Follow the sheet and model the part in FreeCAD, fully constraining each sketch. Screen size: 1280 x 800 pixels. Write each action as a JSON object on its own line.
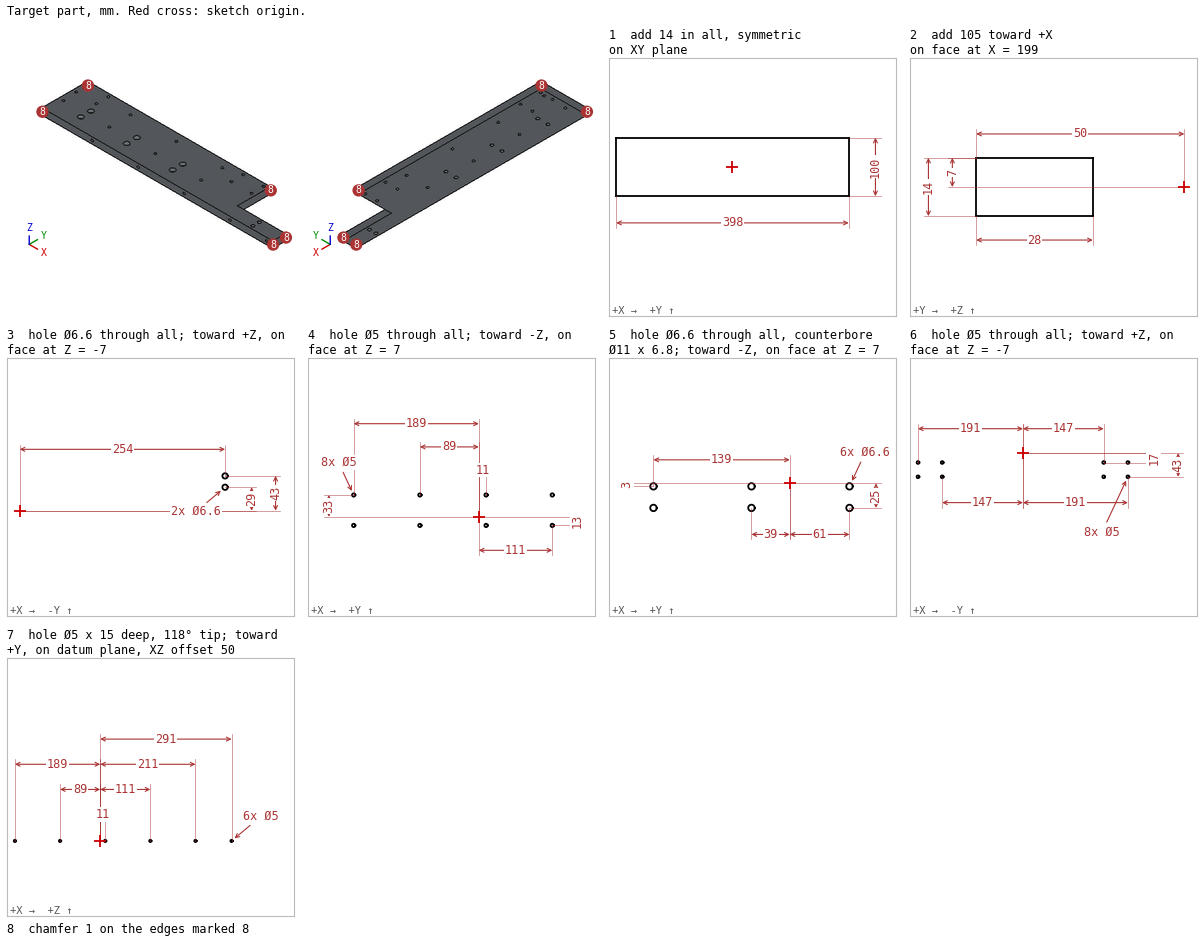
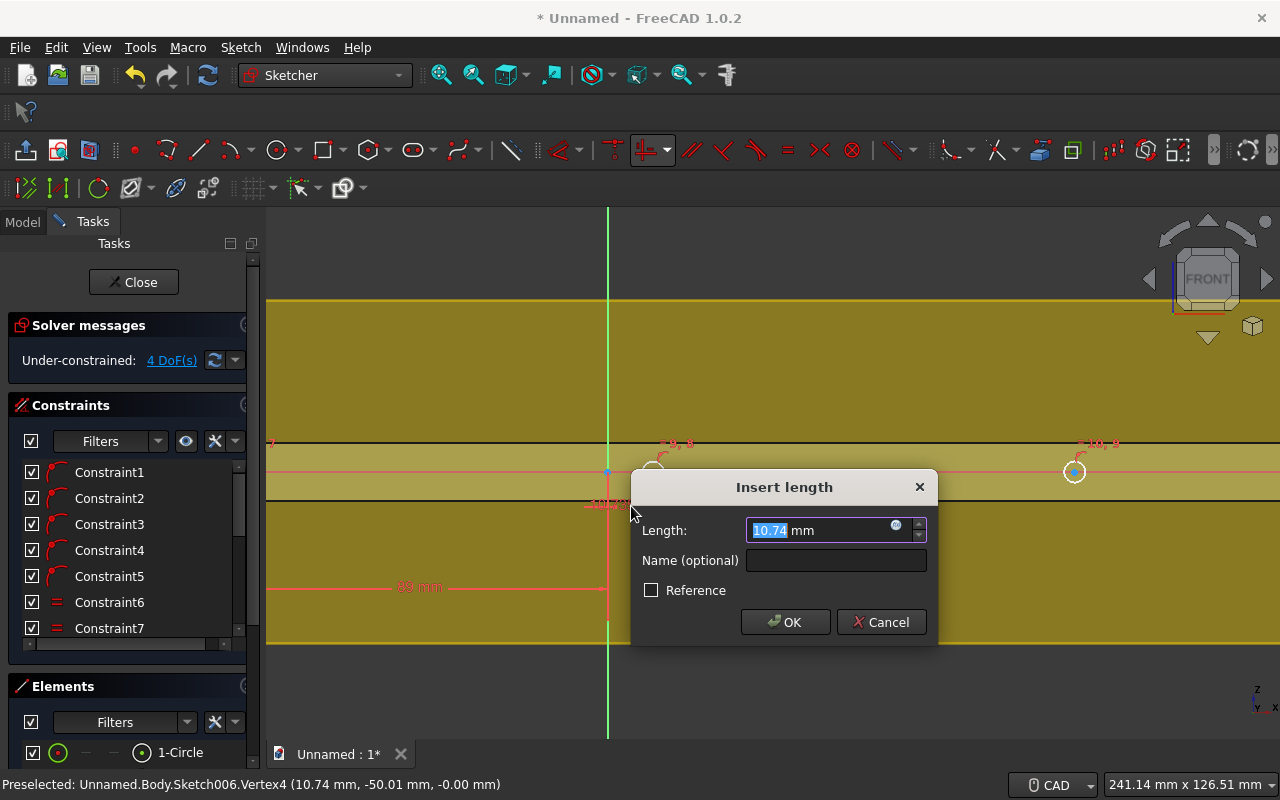
{"action": "type", "text": "11"}
{"action": "key", "text": "Return"}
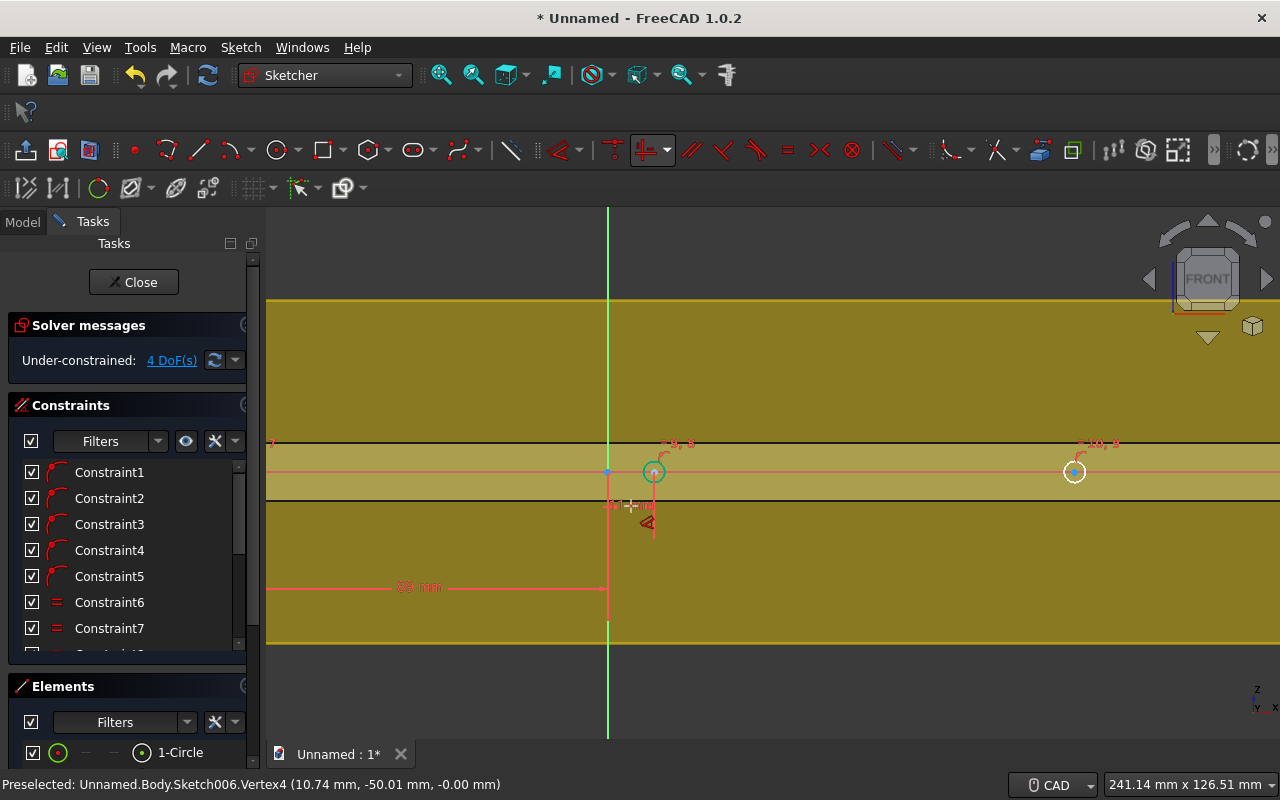
{"action": "scroll", "coordinate": [654, 473], "scroll_direction": "down", "scroll_amount": 6}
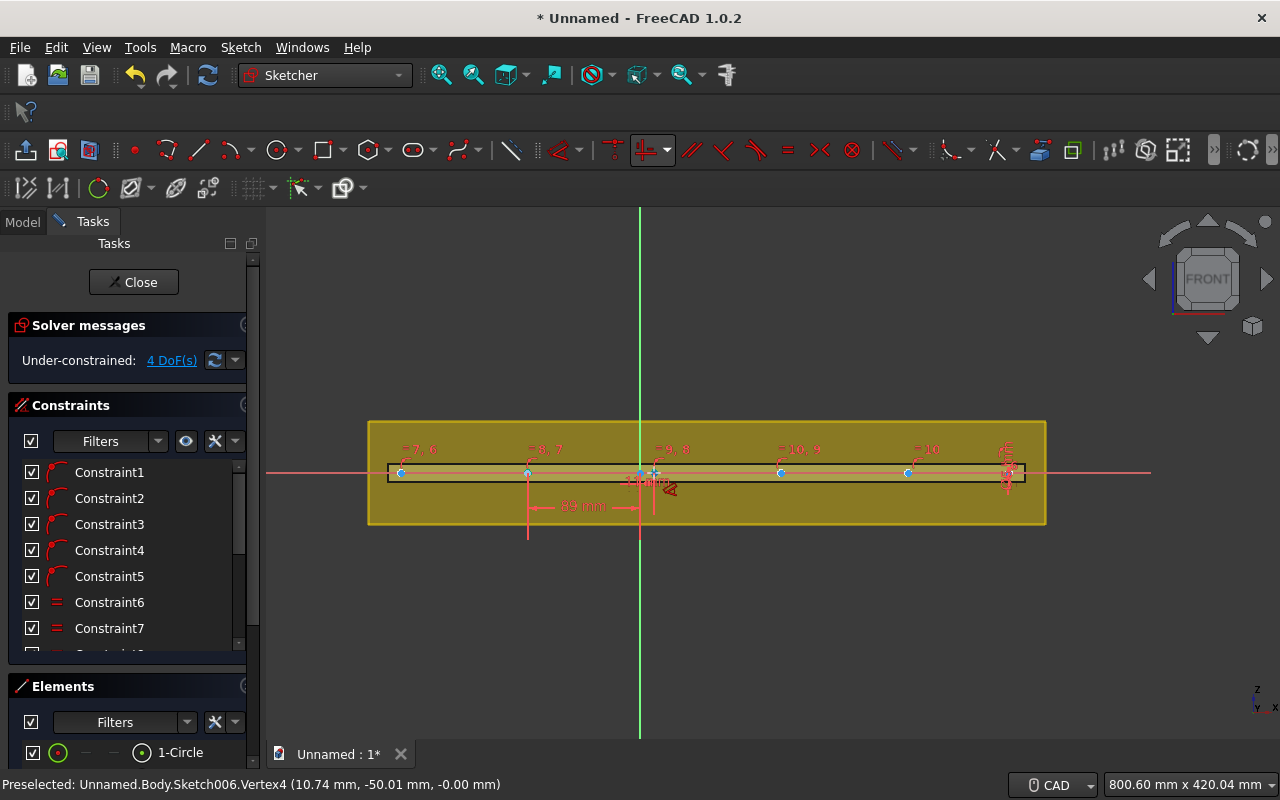
{"action": "left_click", "coordinate": [1009, 473]}
{"action": "left_click", "coordinate": [825, 507]}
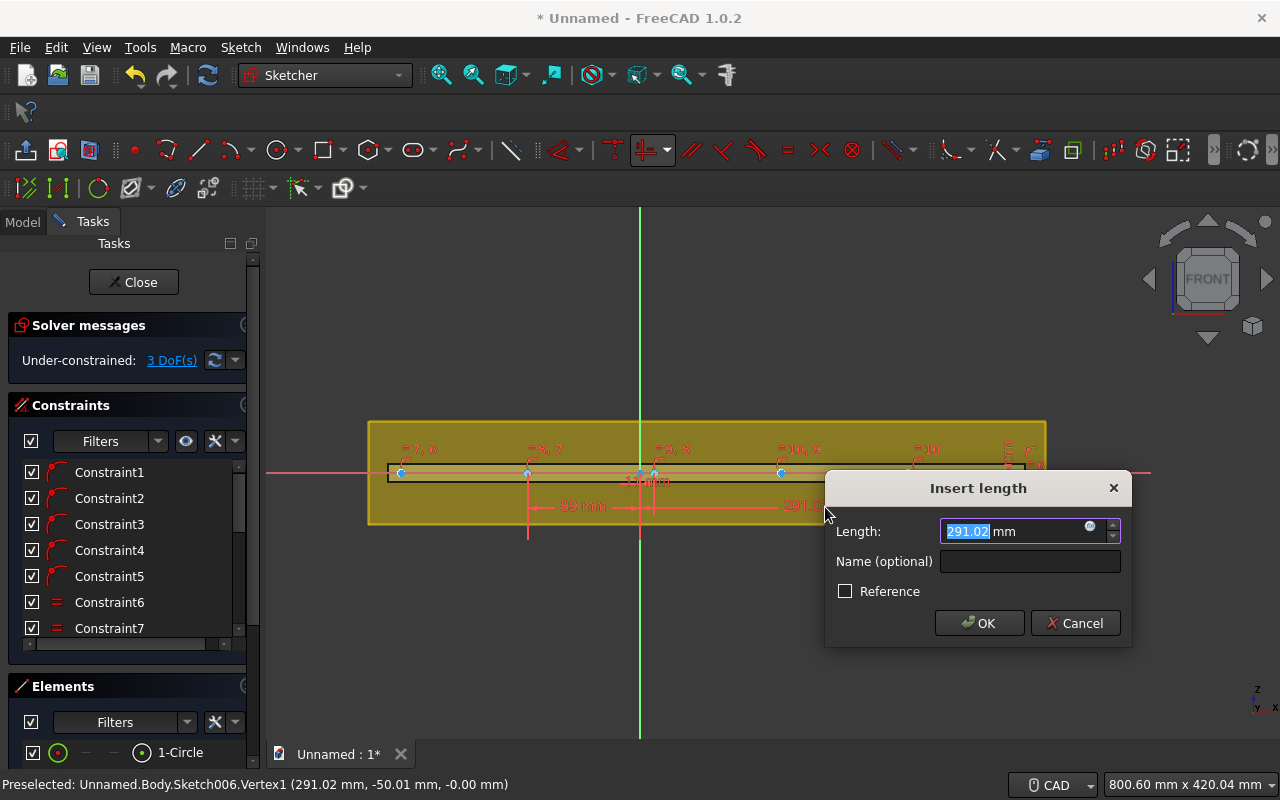
{"action": "type", "text": "291"}
{"action": "key", "text": "Return"}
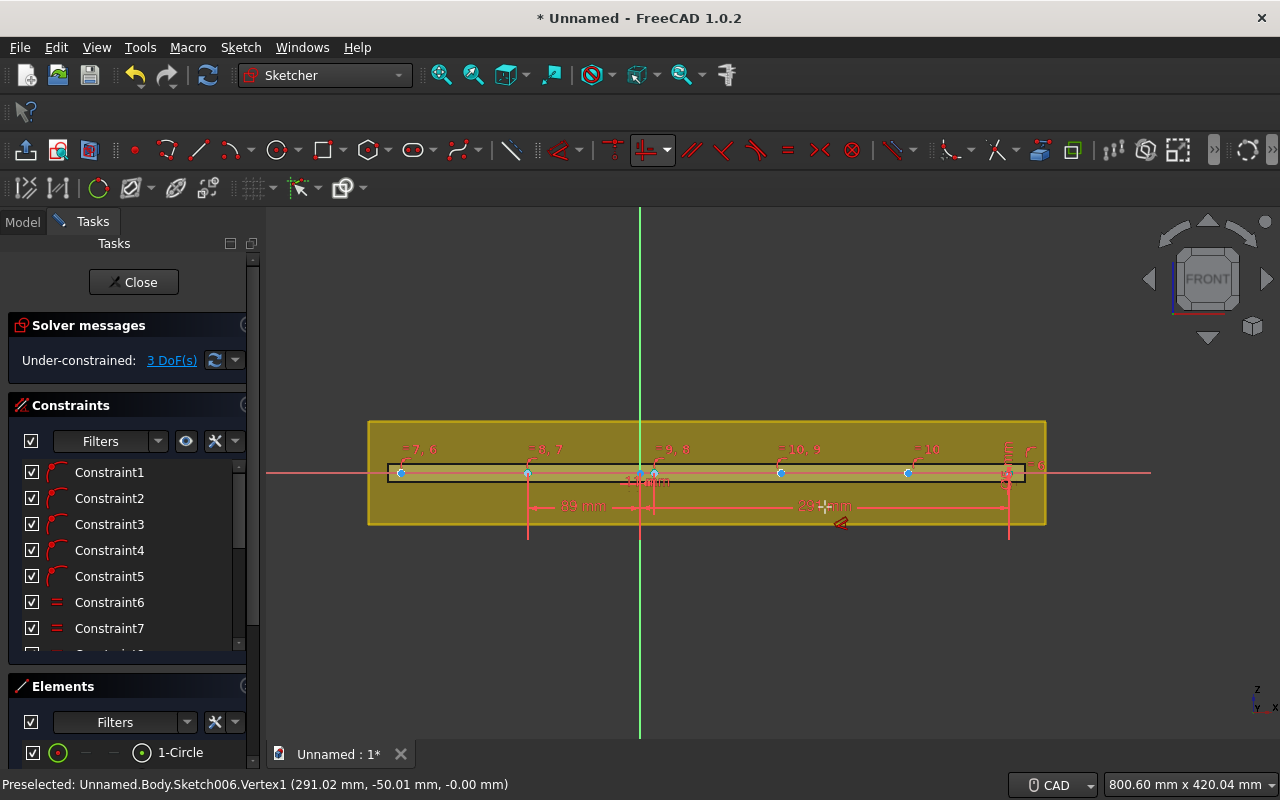
{"action": "left_click", "coordinate": [401, 473]}
{"action": "left_click", "coordinate": [466, 507]}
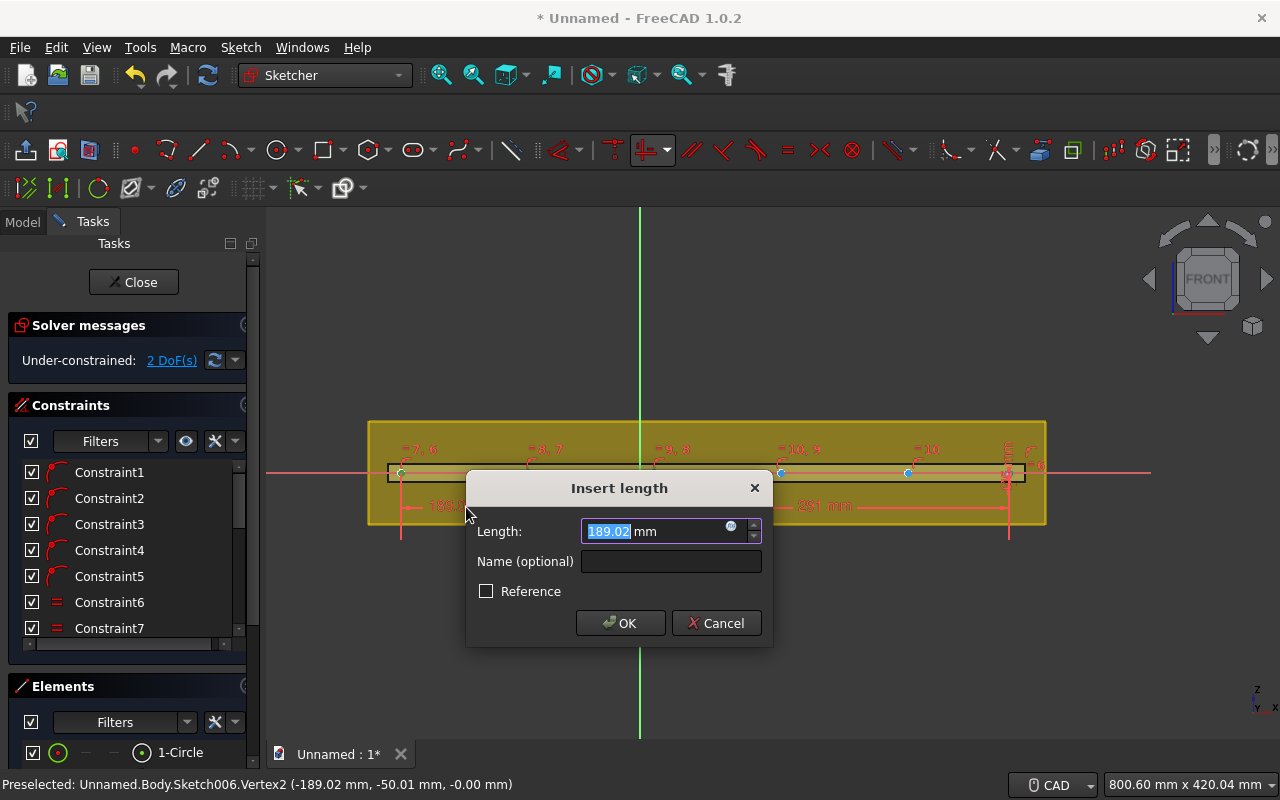
{"action": "type", "text": "189"}
{"action": "key", "text": "Return"}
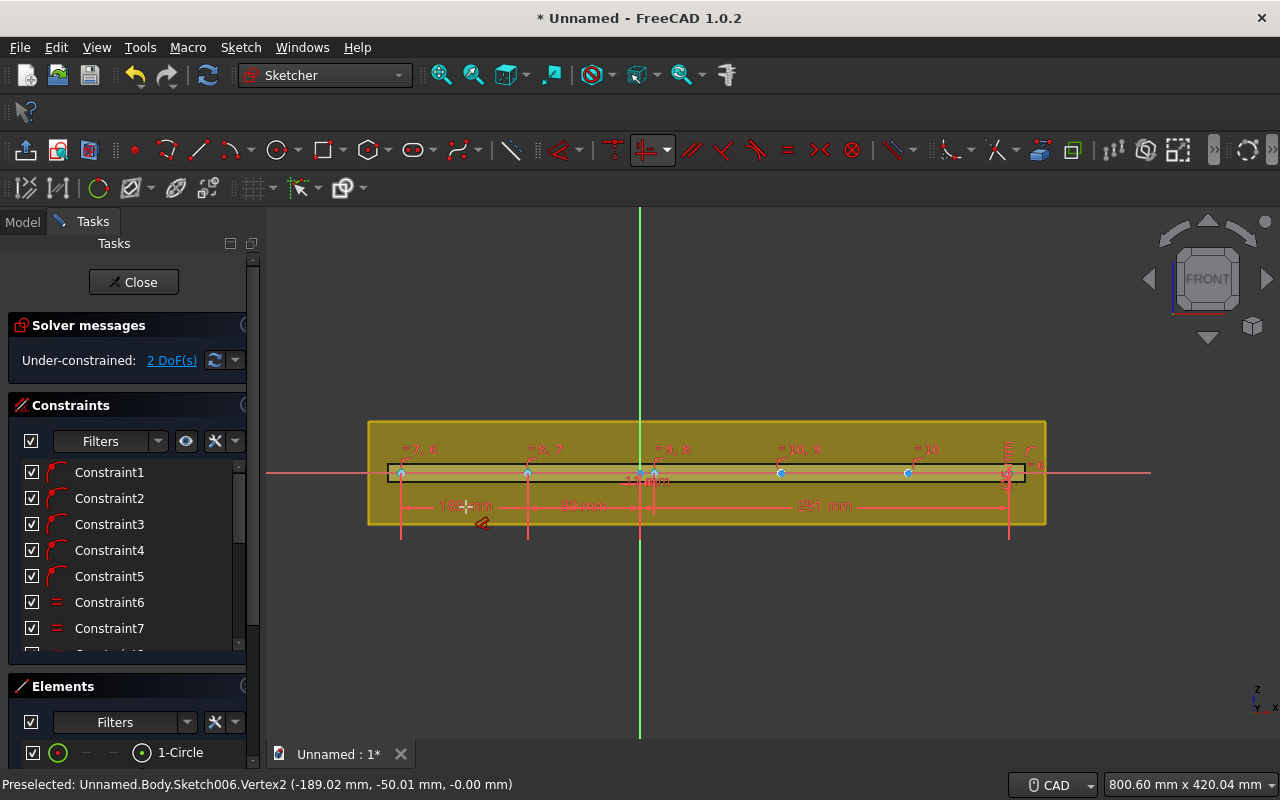
{"action": "left_click", "coordinate": [781, 473]}
{"action": "left_click", "coordinate": [711, 507]}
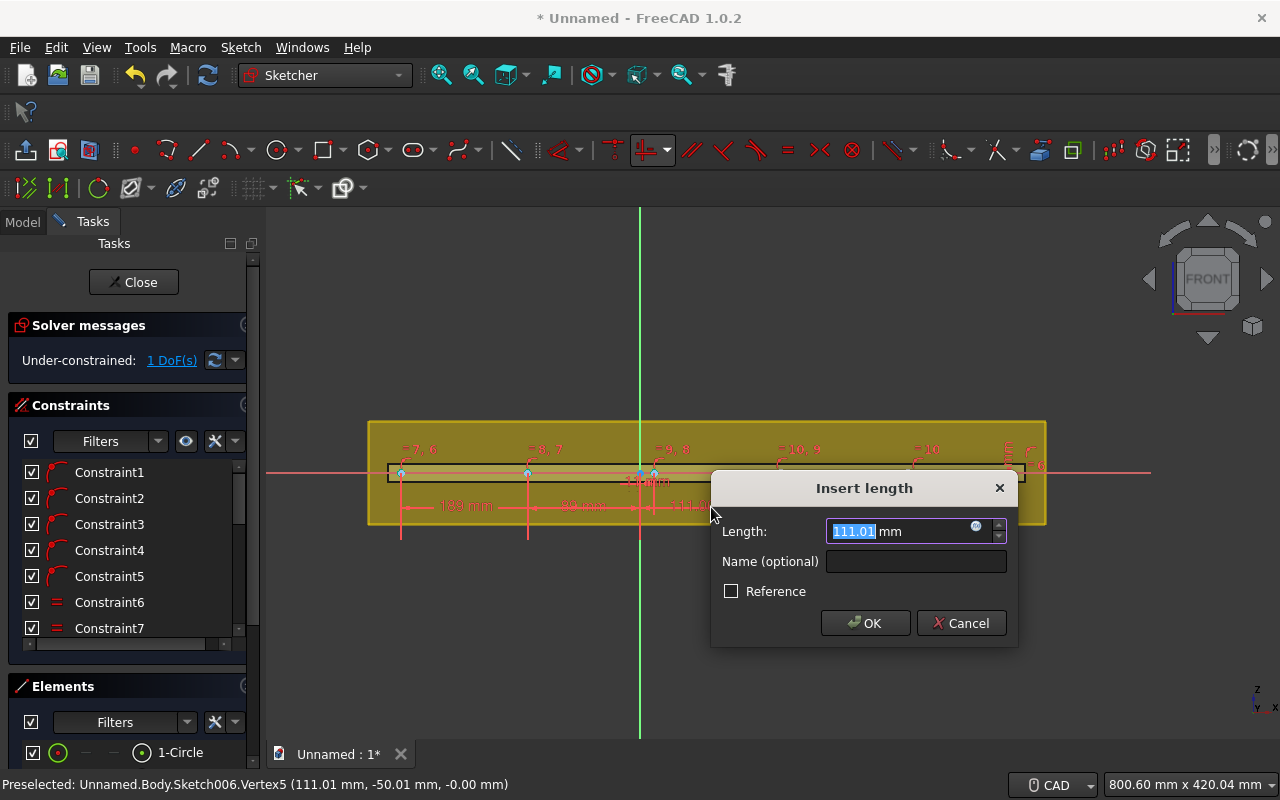
{"action": "type", "text": "111"}
{"action": "key", "text": "Return"}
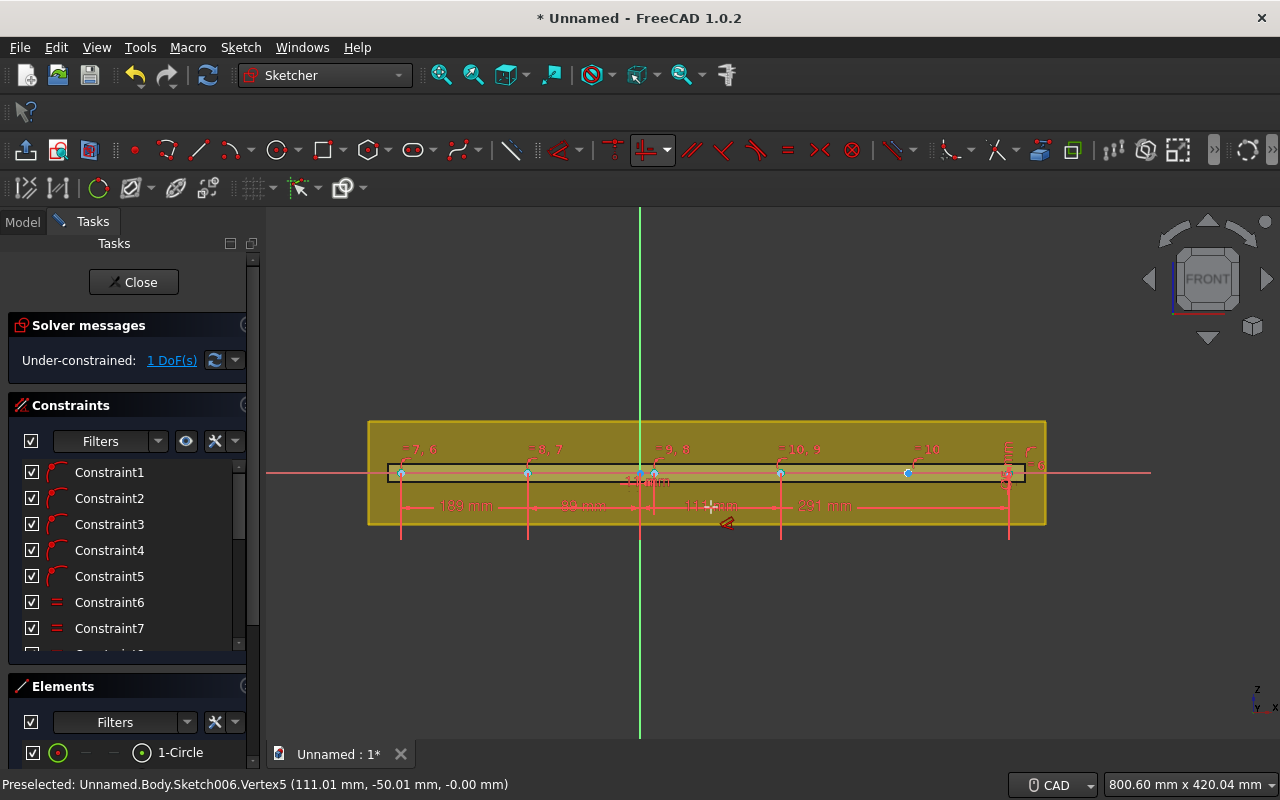
{"action": "left_click", "coordinate": [908, 473]}
{"action": "left_click", "coordinate": [774, 439]}